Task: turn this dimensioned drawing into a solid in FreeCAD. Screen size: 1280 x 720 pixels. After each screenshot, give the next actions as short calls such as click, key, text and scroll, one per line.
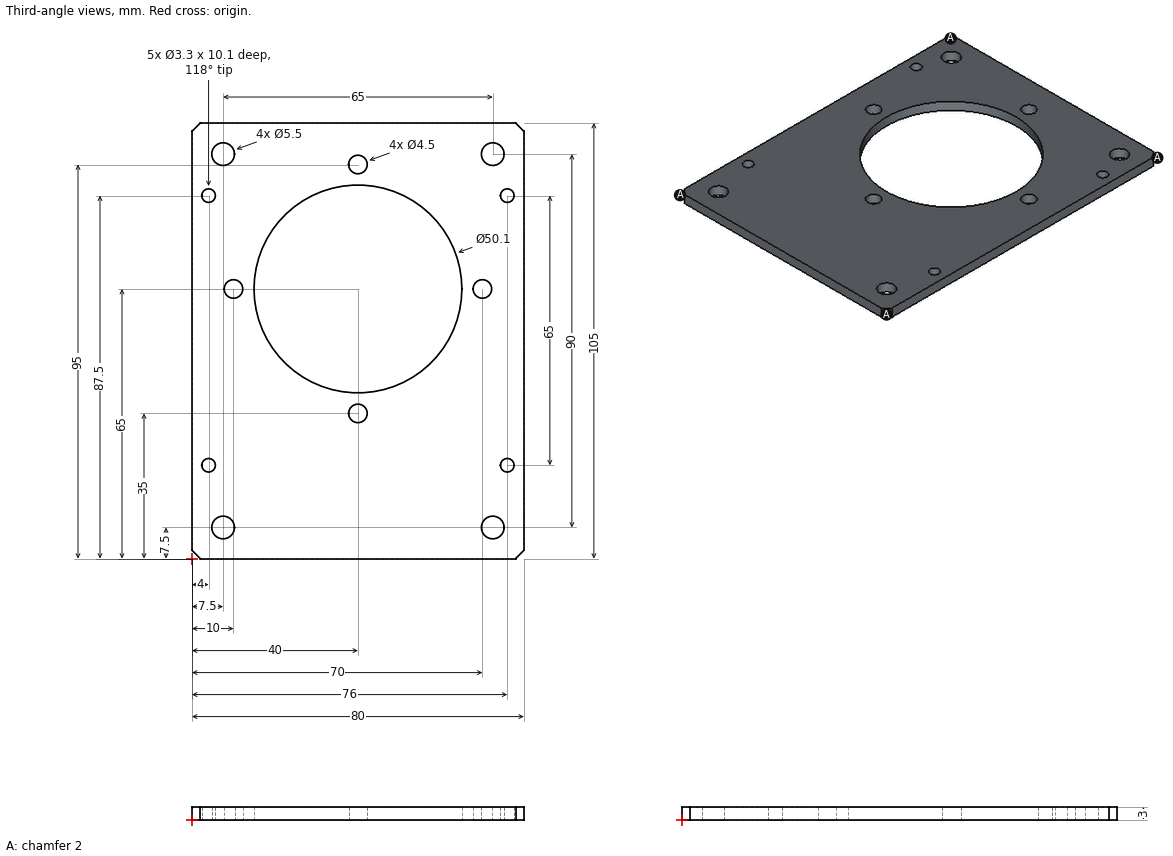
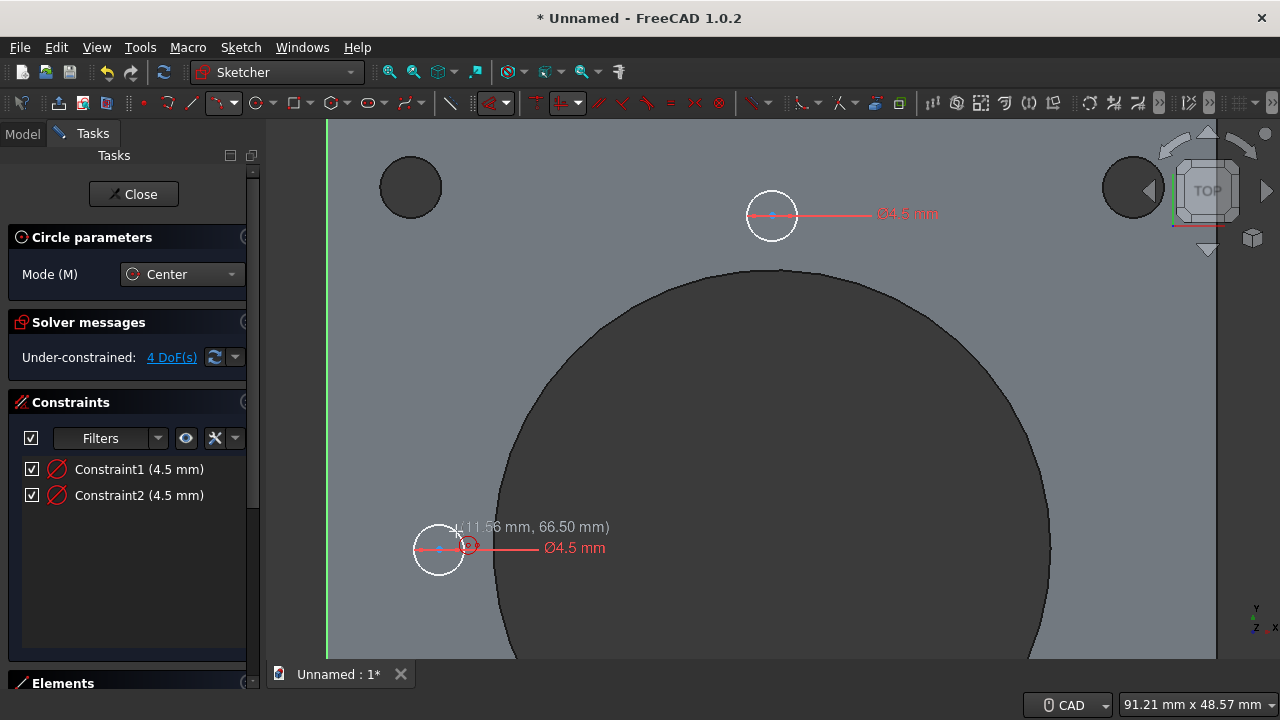
click(1106, 549)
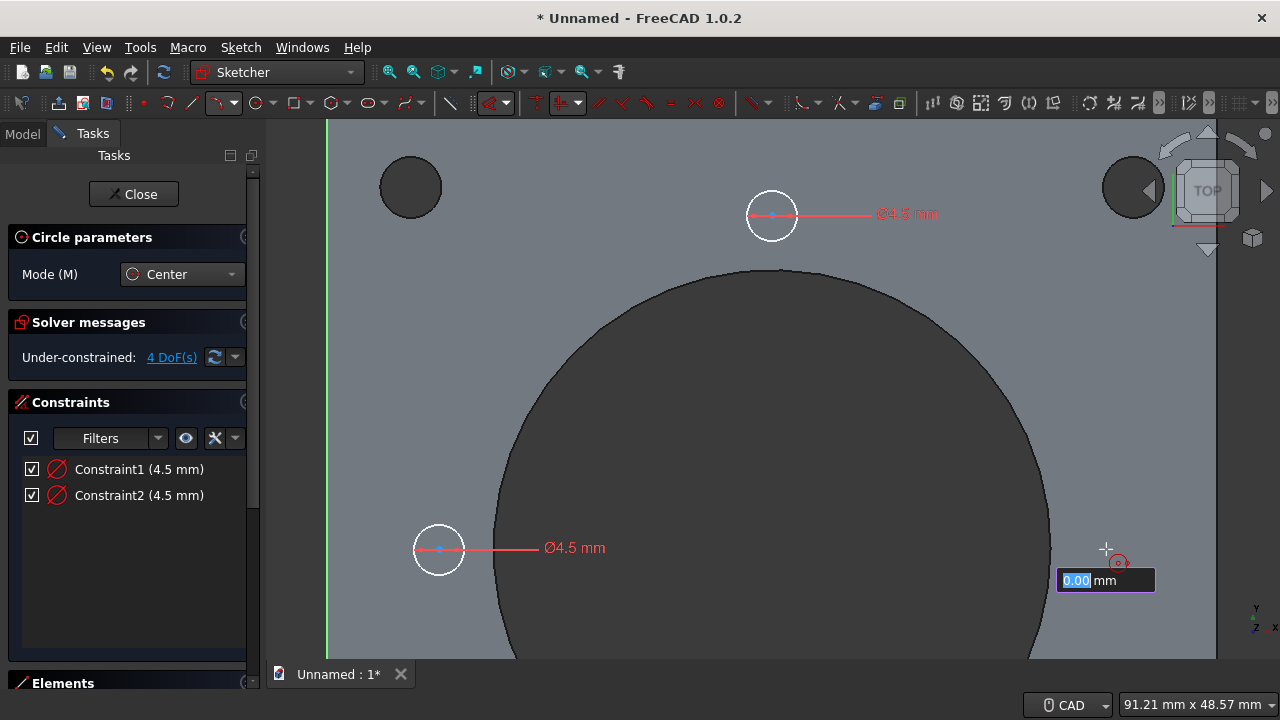
scroll(694, 242, down, 6)
move(824, 329)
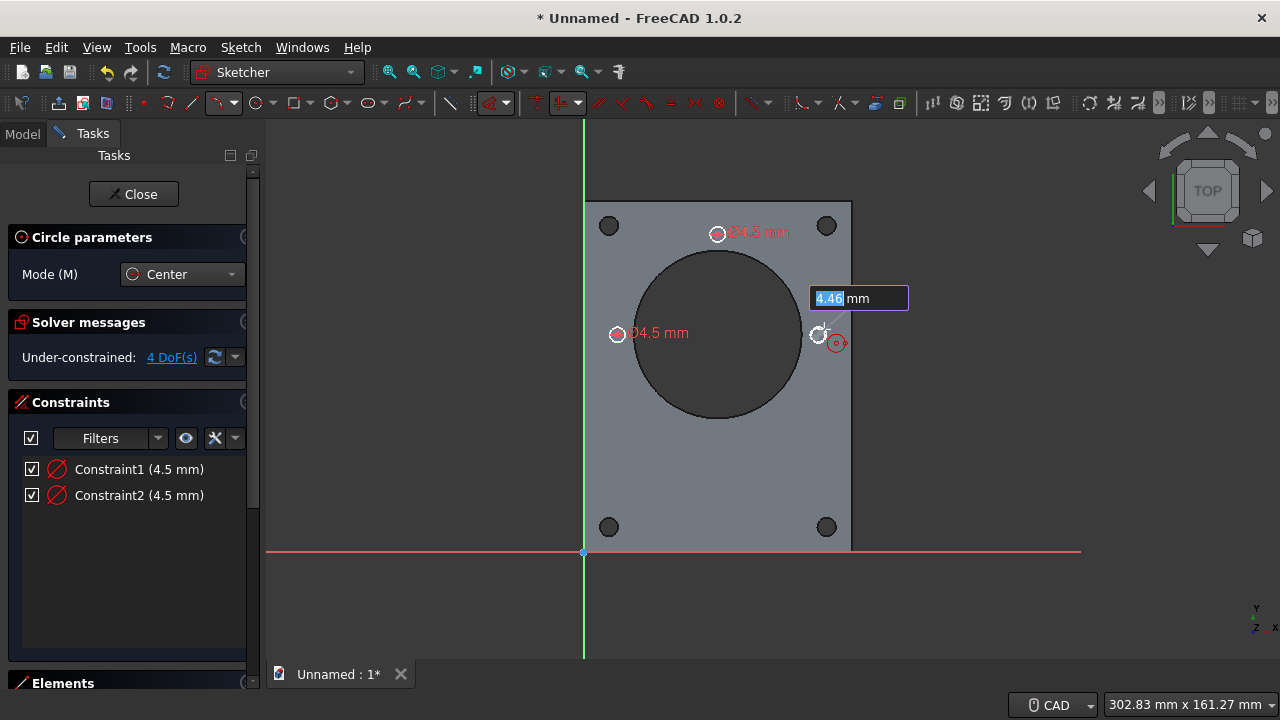
text(4.5)
key(Return)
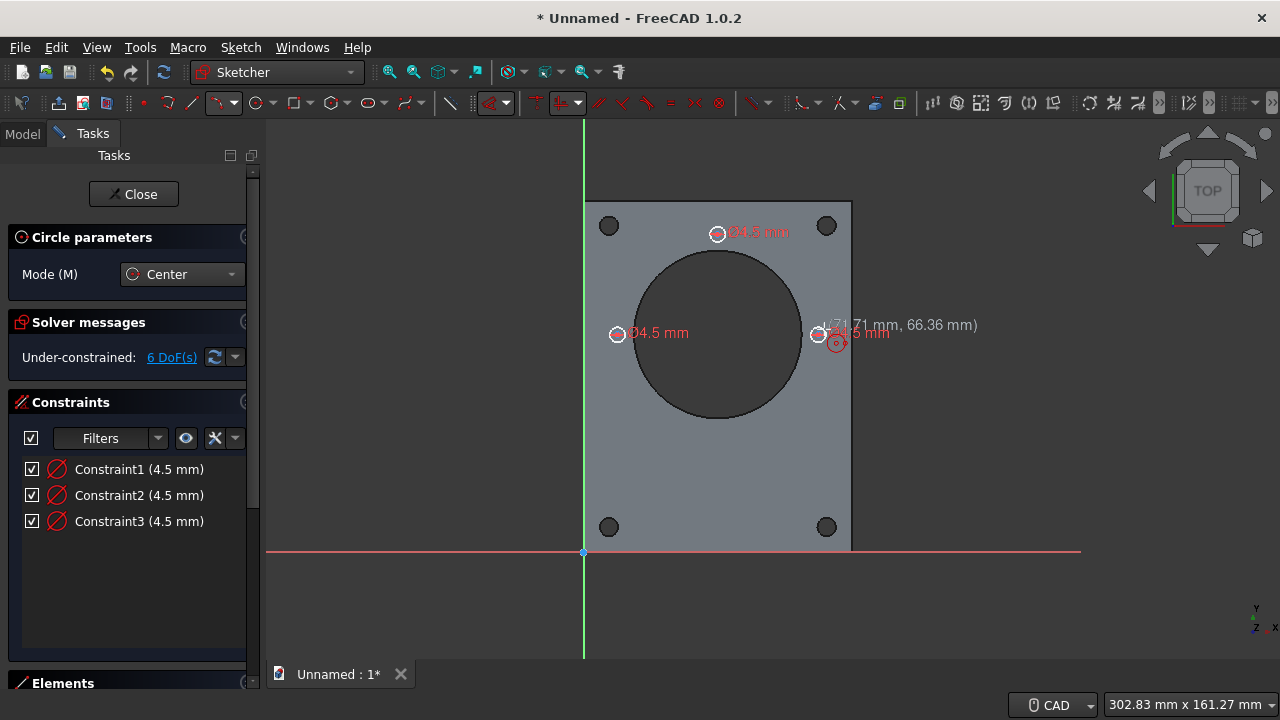
scroll(718, 435, up, 6)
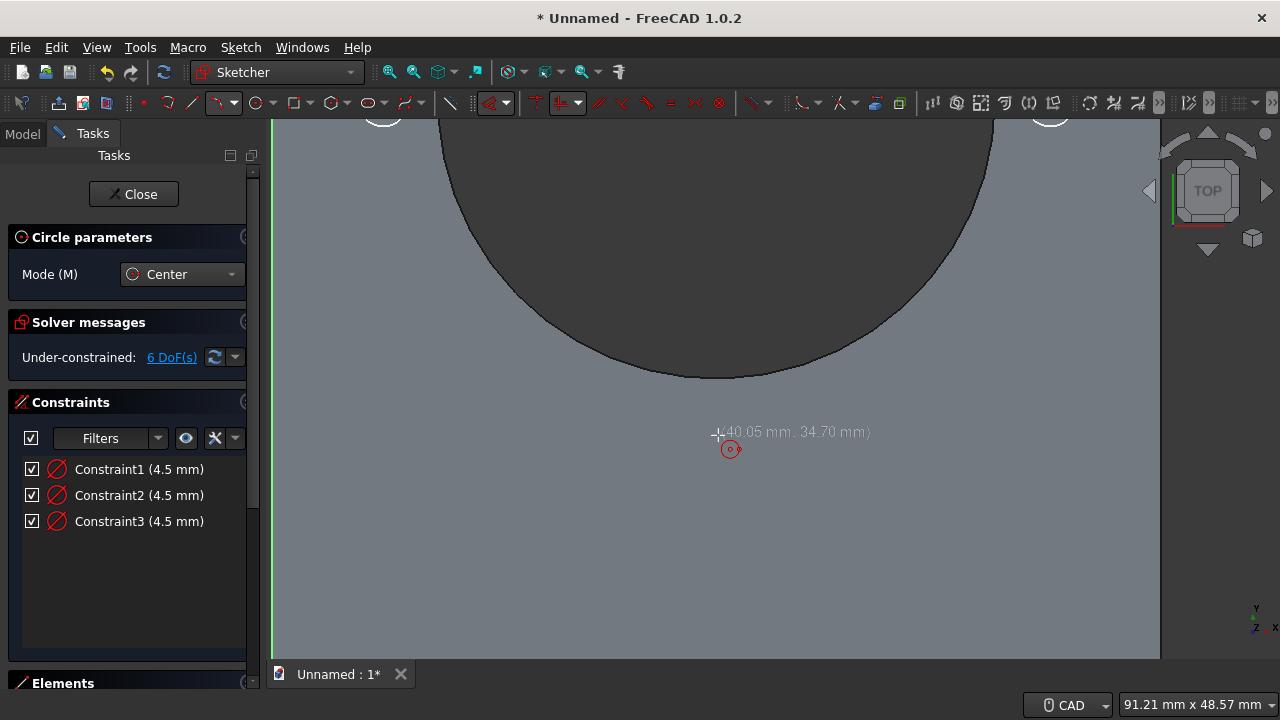
click(716, 434)
move(734, 416)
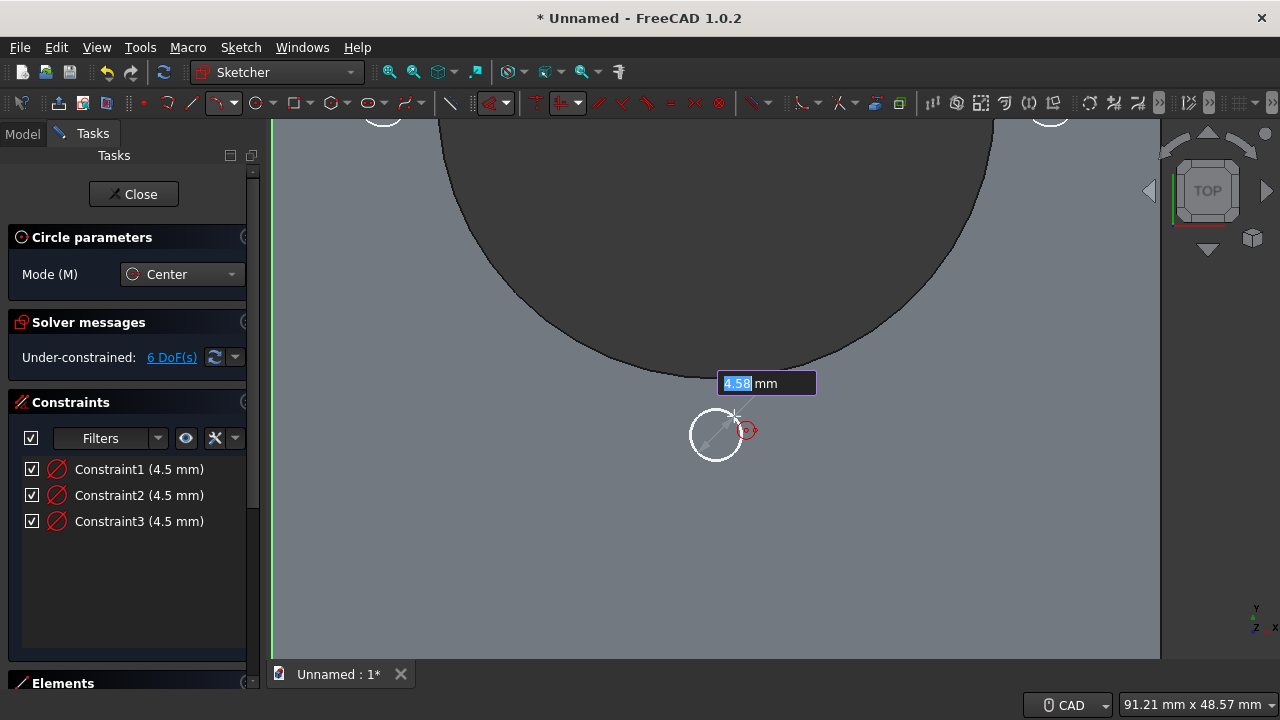
text(4.5)
key(Return)
key(Escape)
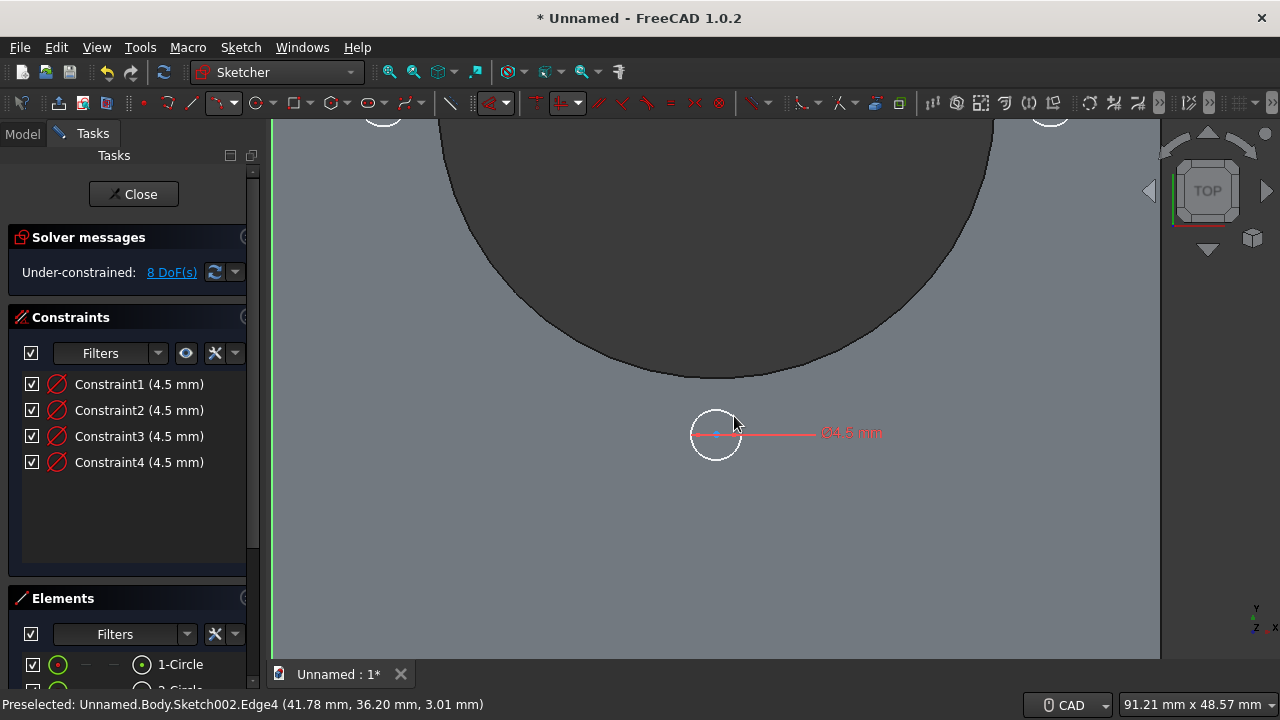
scroll(718, 435, down, 6)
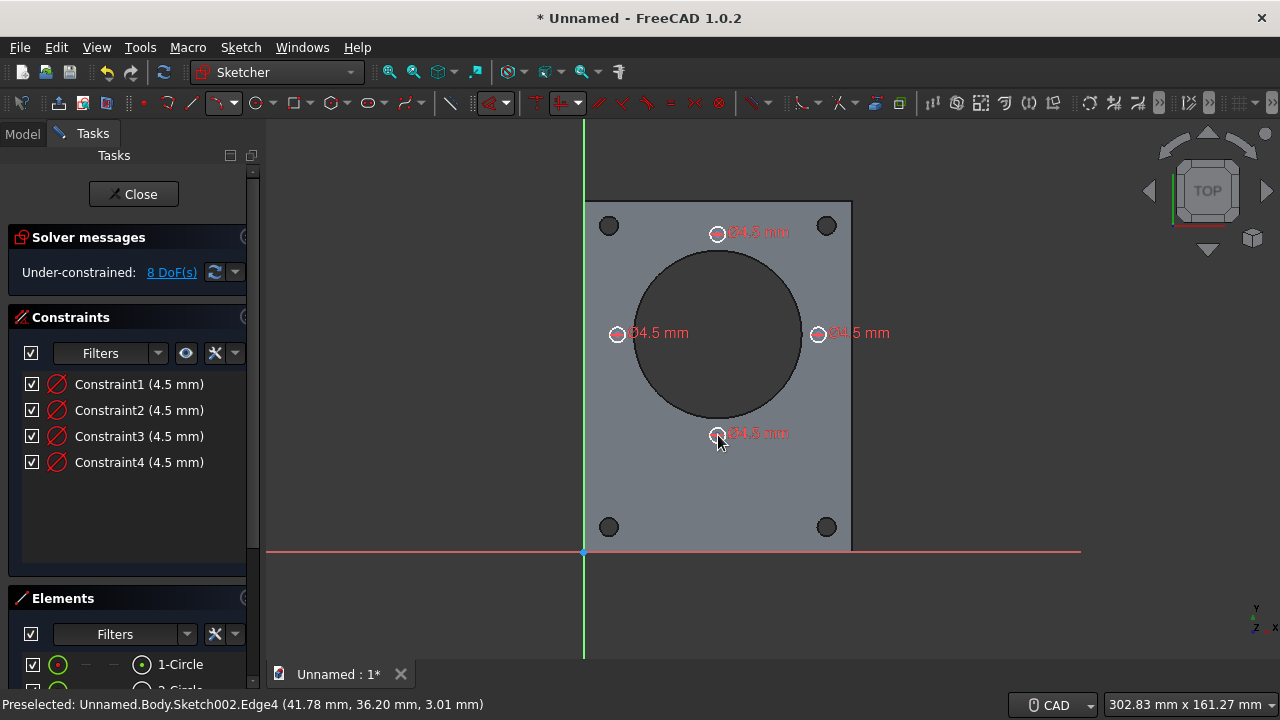
click(617, 335)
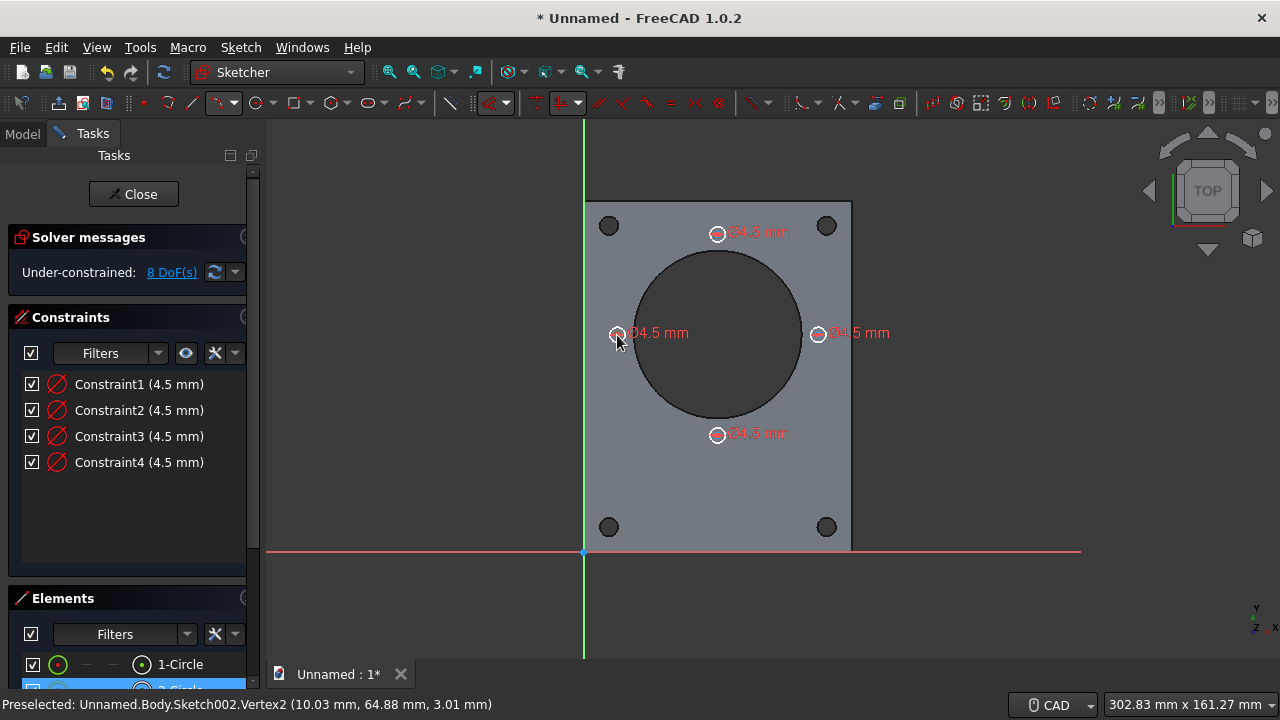
click(818, 335)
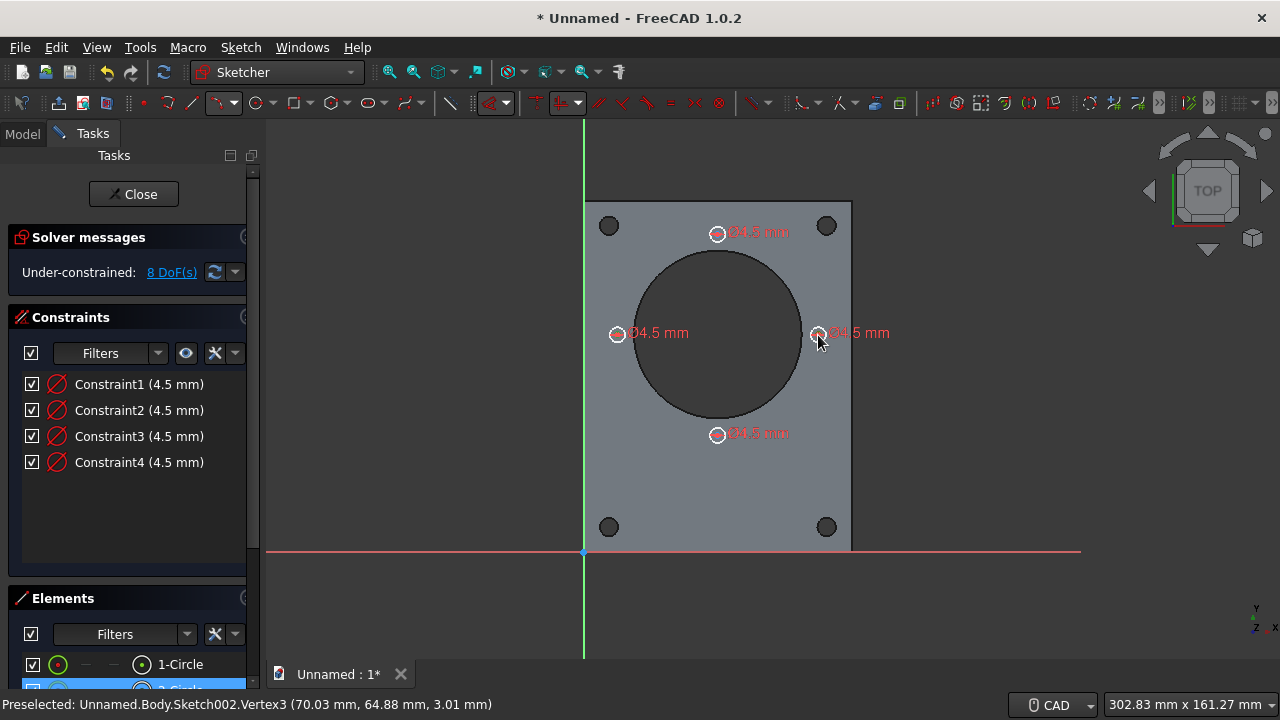
click(580, 104)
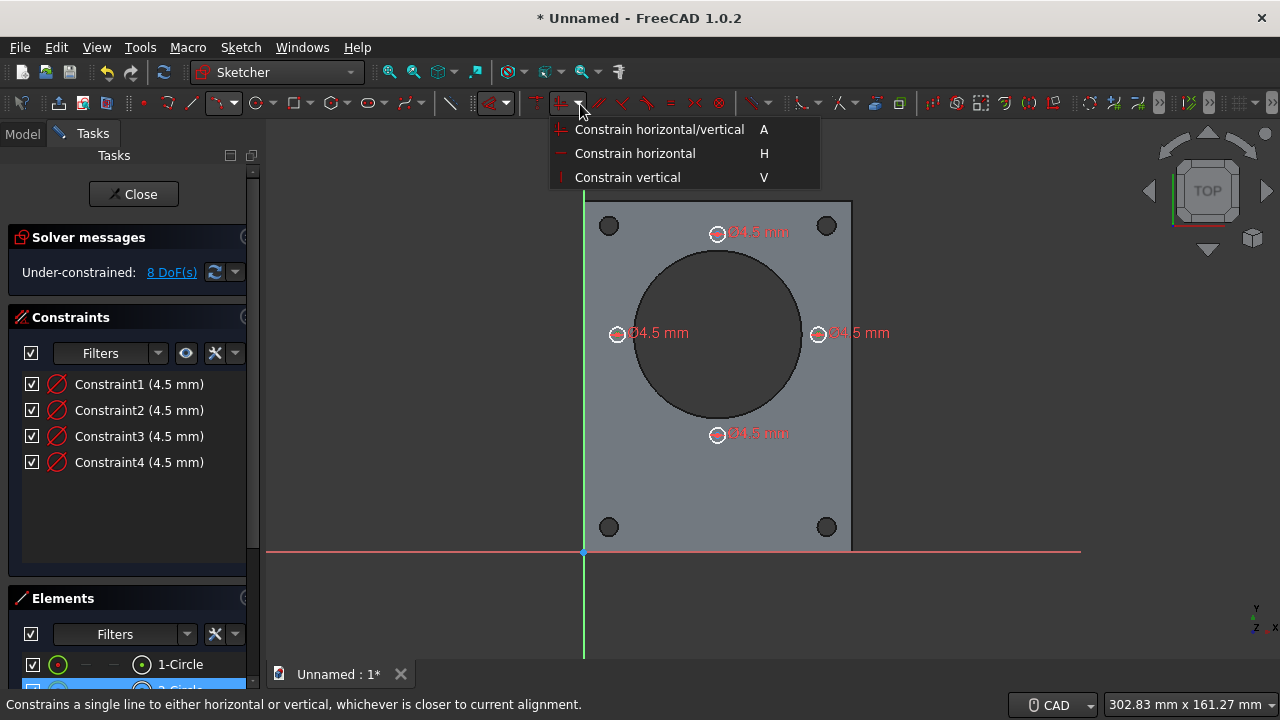
click(685, 153)